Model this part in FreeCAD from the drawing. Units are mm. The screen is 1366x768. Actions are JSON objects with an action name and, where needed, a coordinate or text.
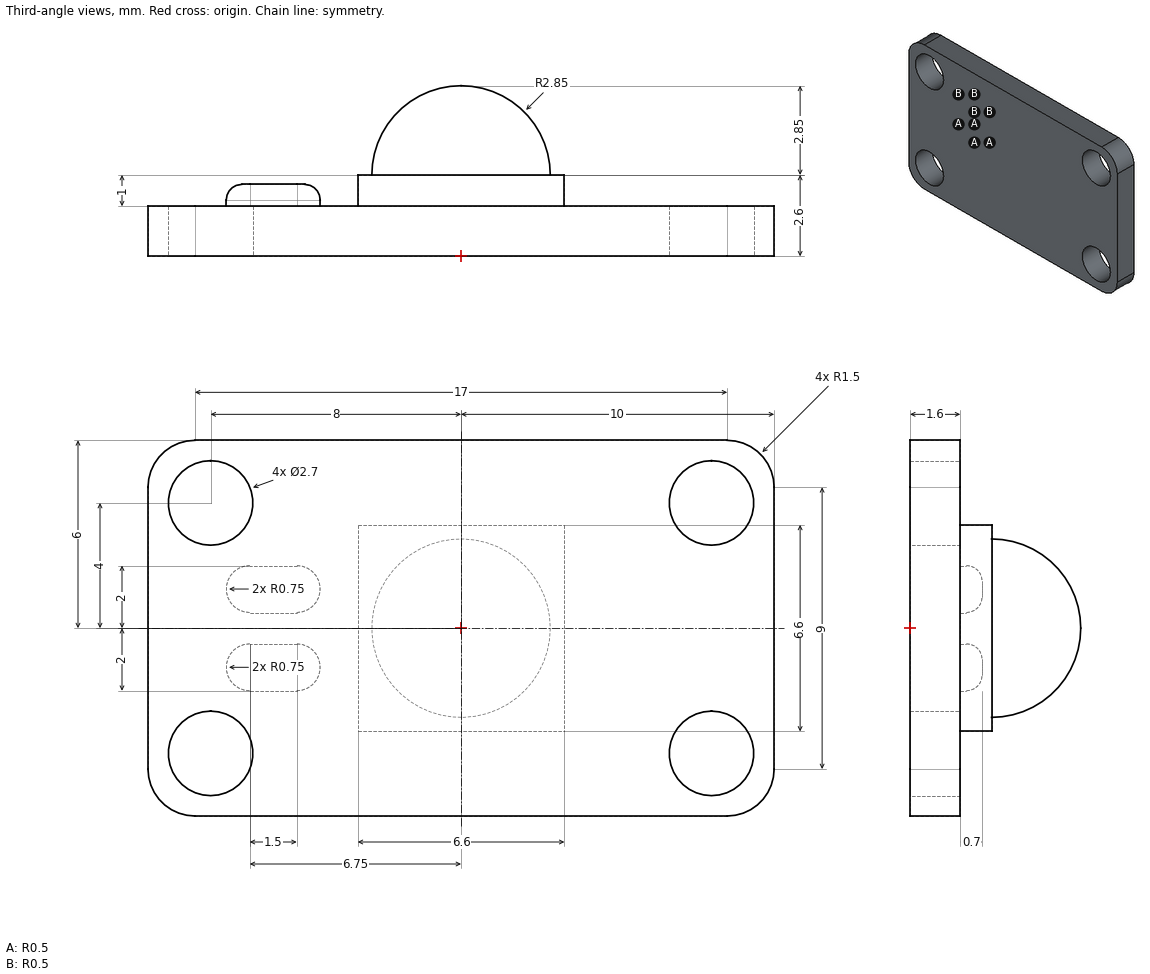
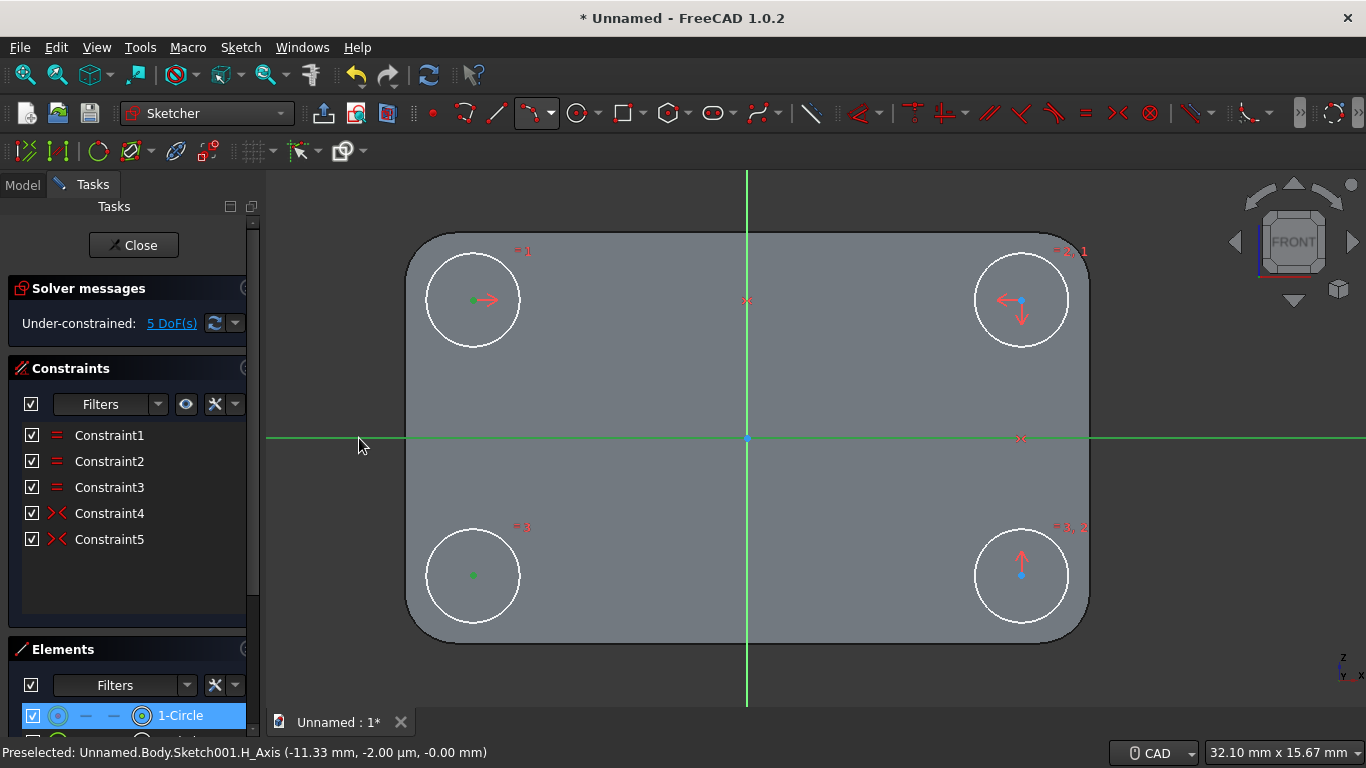
{"action": "left_click", "coordinate": [1118, 114]}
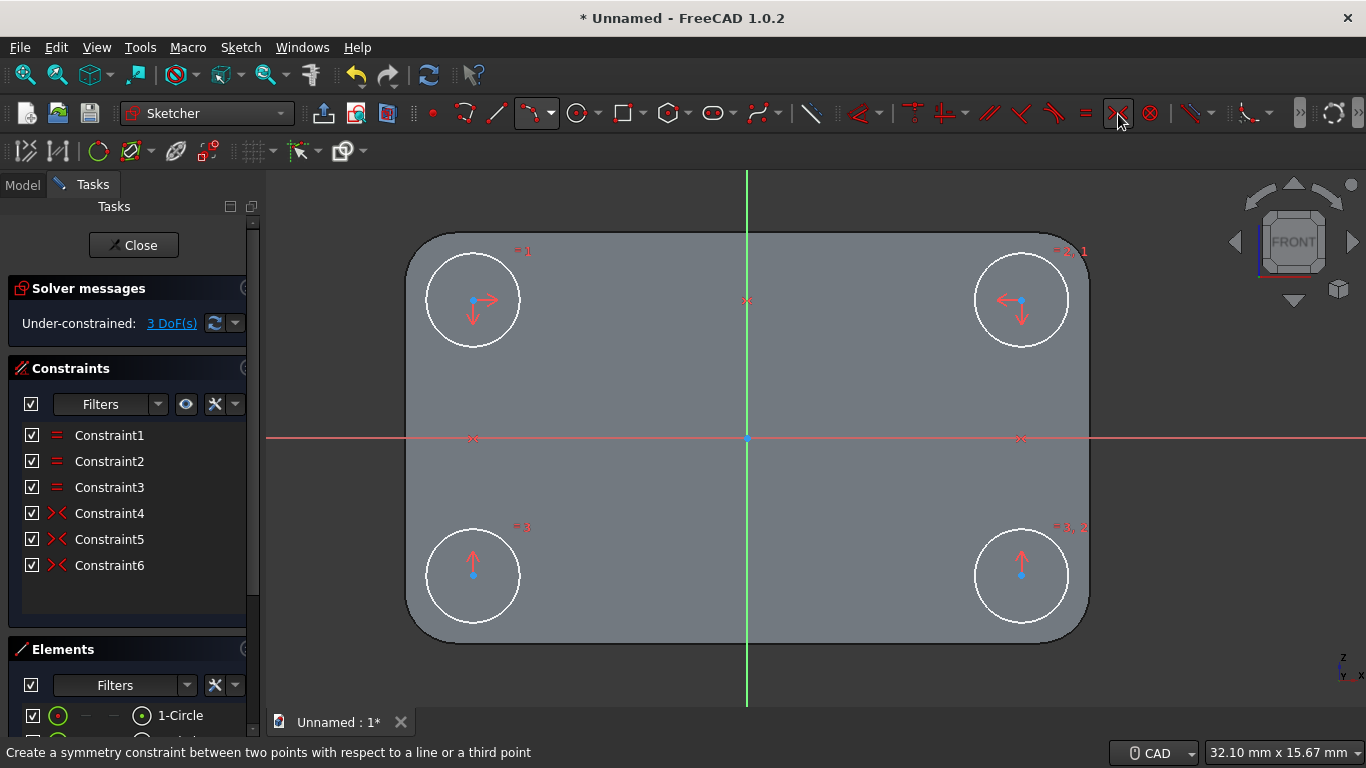
{"action": "left_click", "coordinate": [858, 114]}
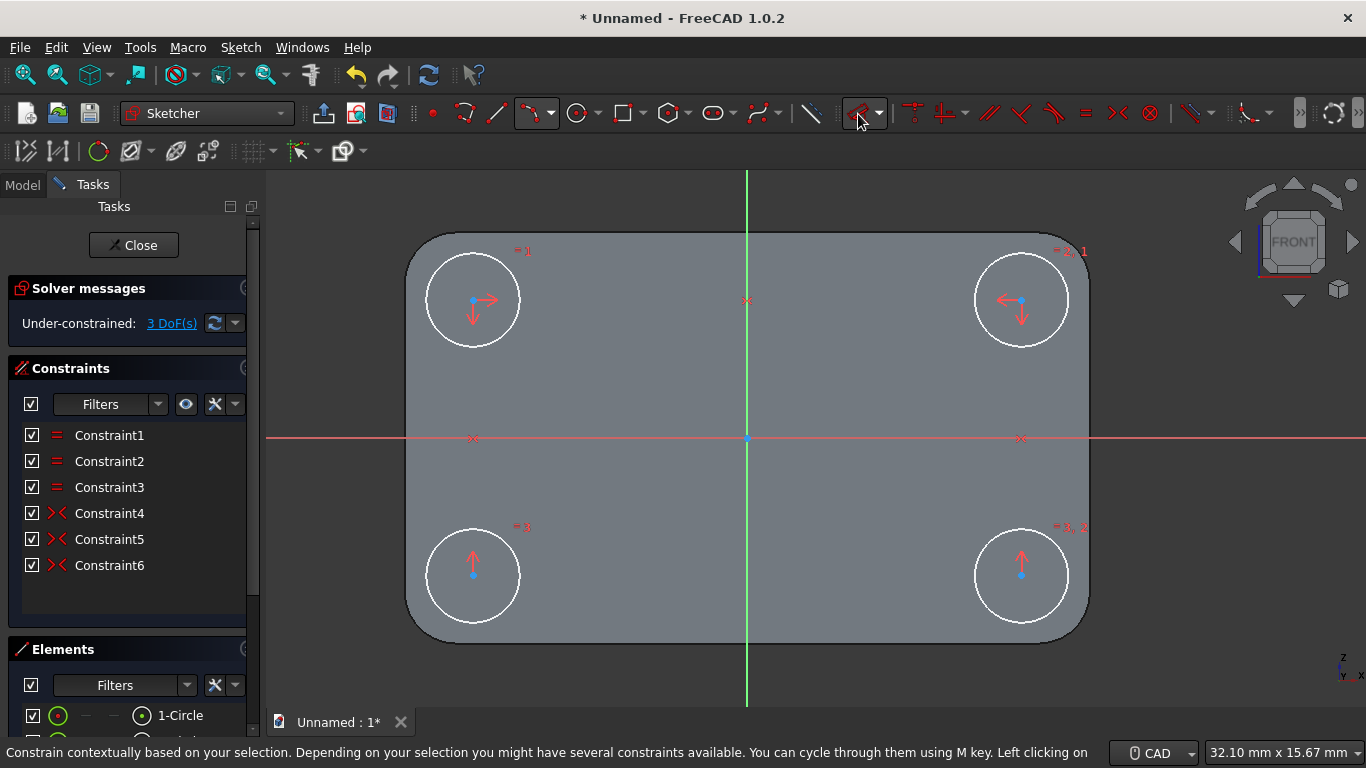
{"action": "left_click", "coordinate": [506, 267]}
{"action": "left_click", "coordinate": [529, 244]}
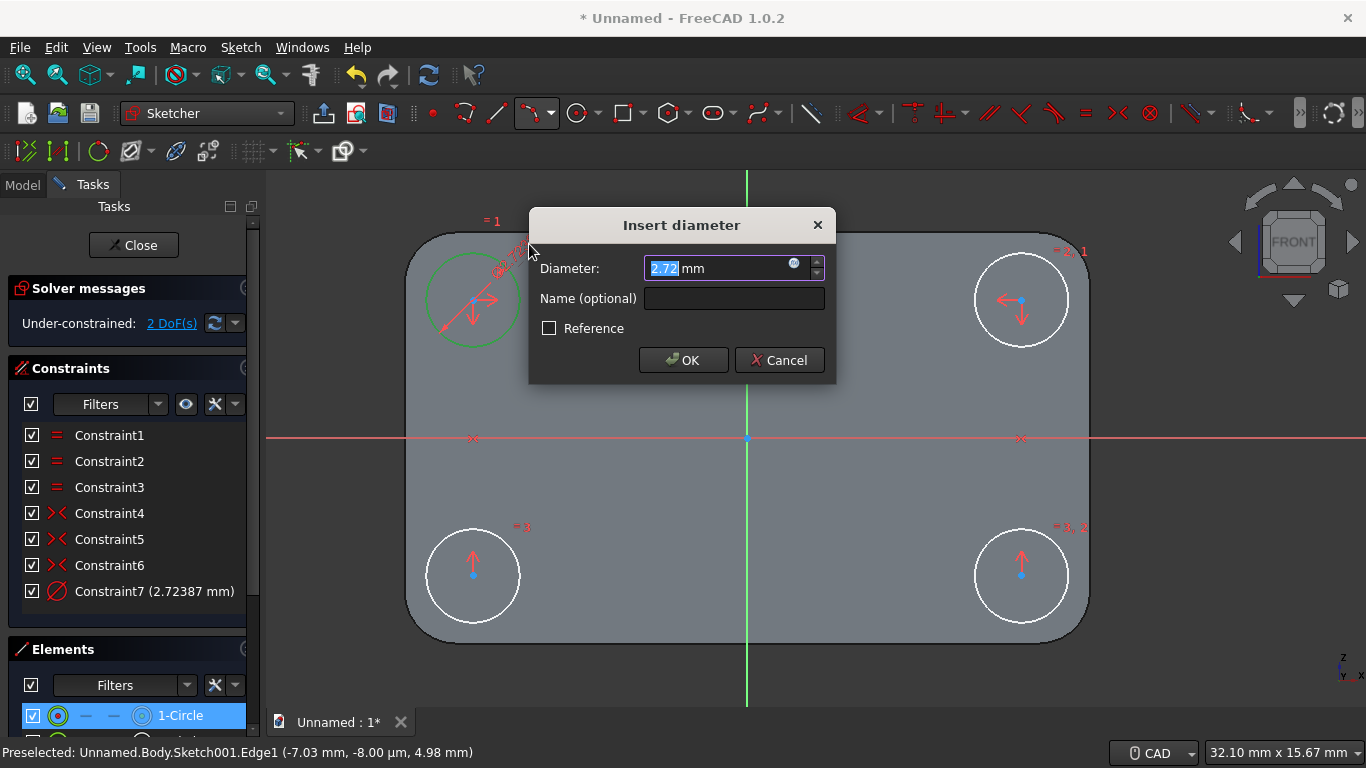
{"action": "type", "text": "2.7"}
{"action": "key", "text": "Return"}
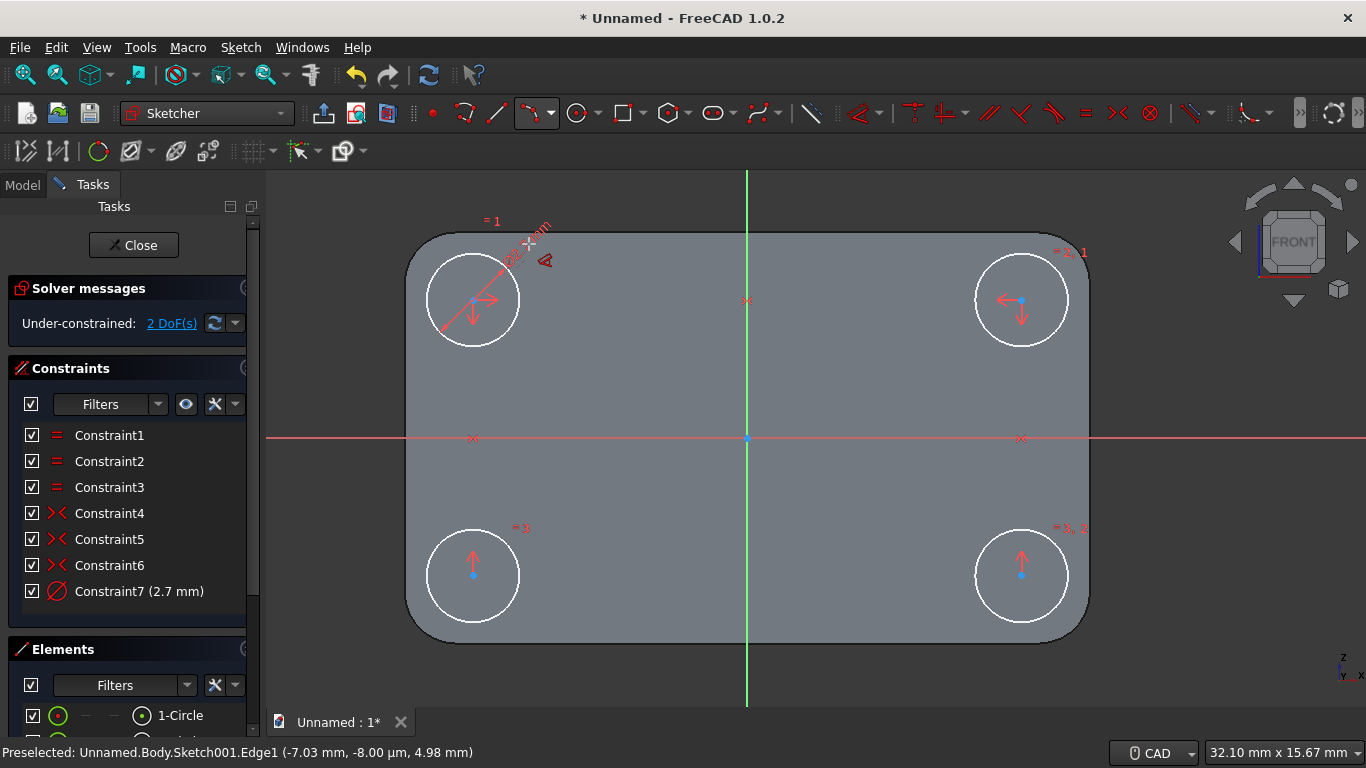
{"action": "left_click", "coordinate": [473, 300]}
{"action": "left_click", "coordinate": [610, 266]}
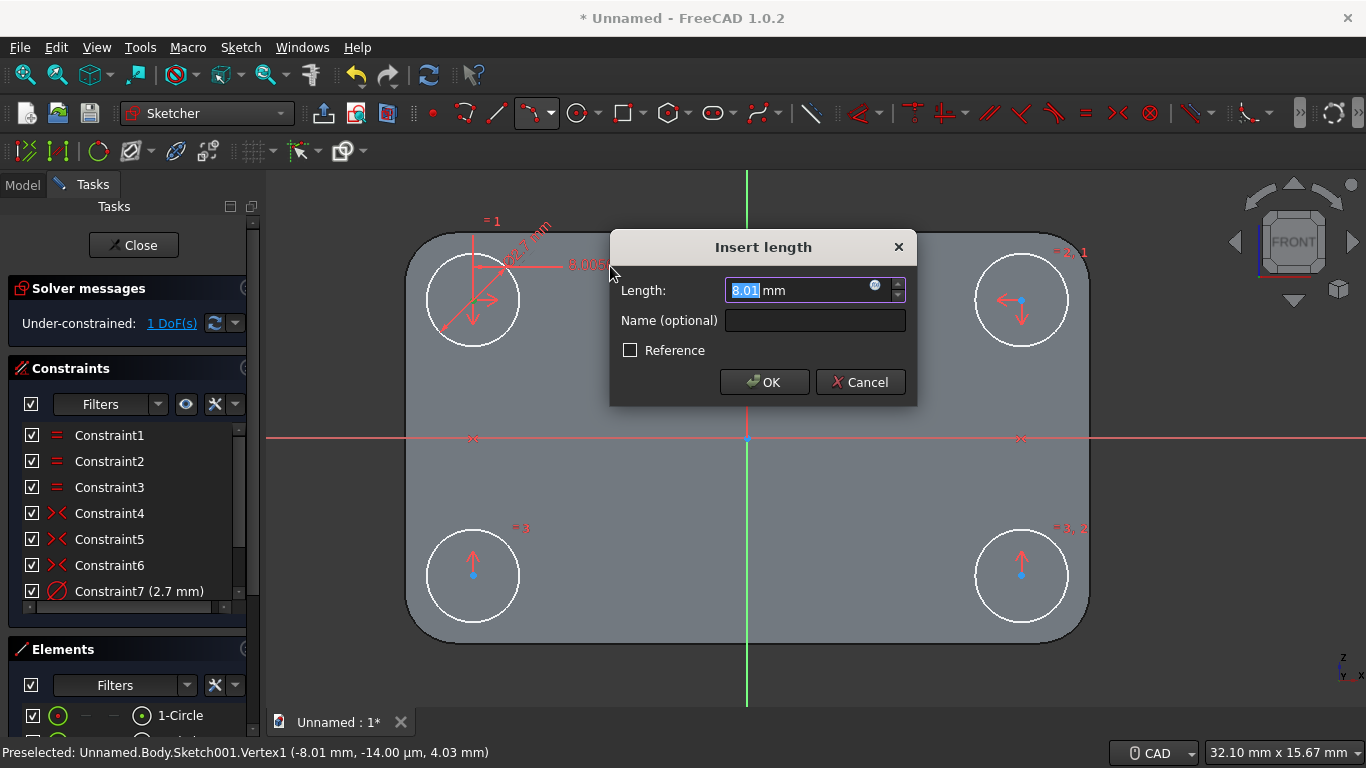
{"action": "type", "text": "8"}
{"action": "key", "text": "Return"}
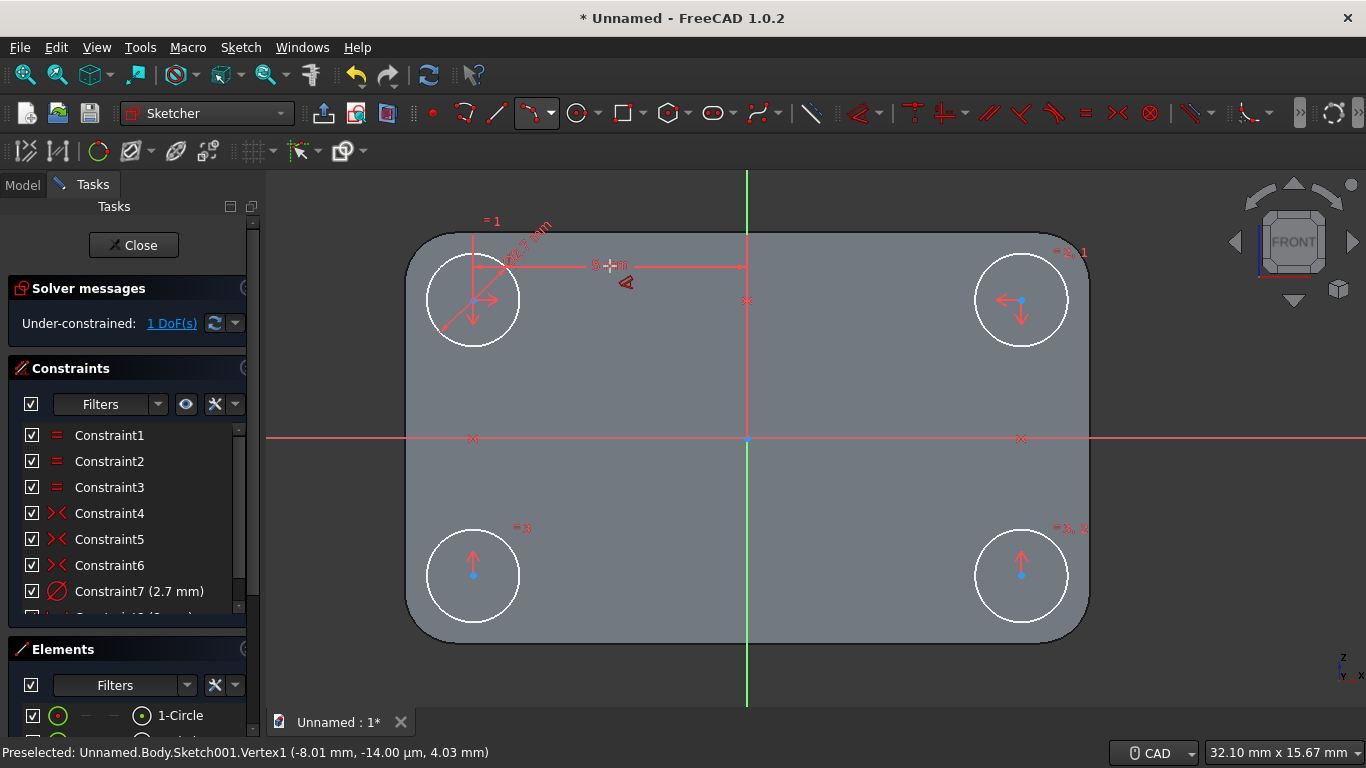
{"action": "left_click", "coordinate": [473, 300]}
{"action": "left_click", "coordinate": [439, 369]}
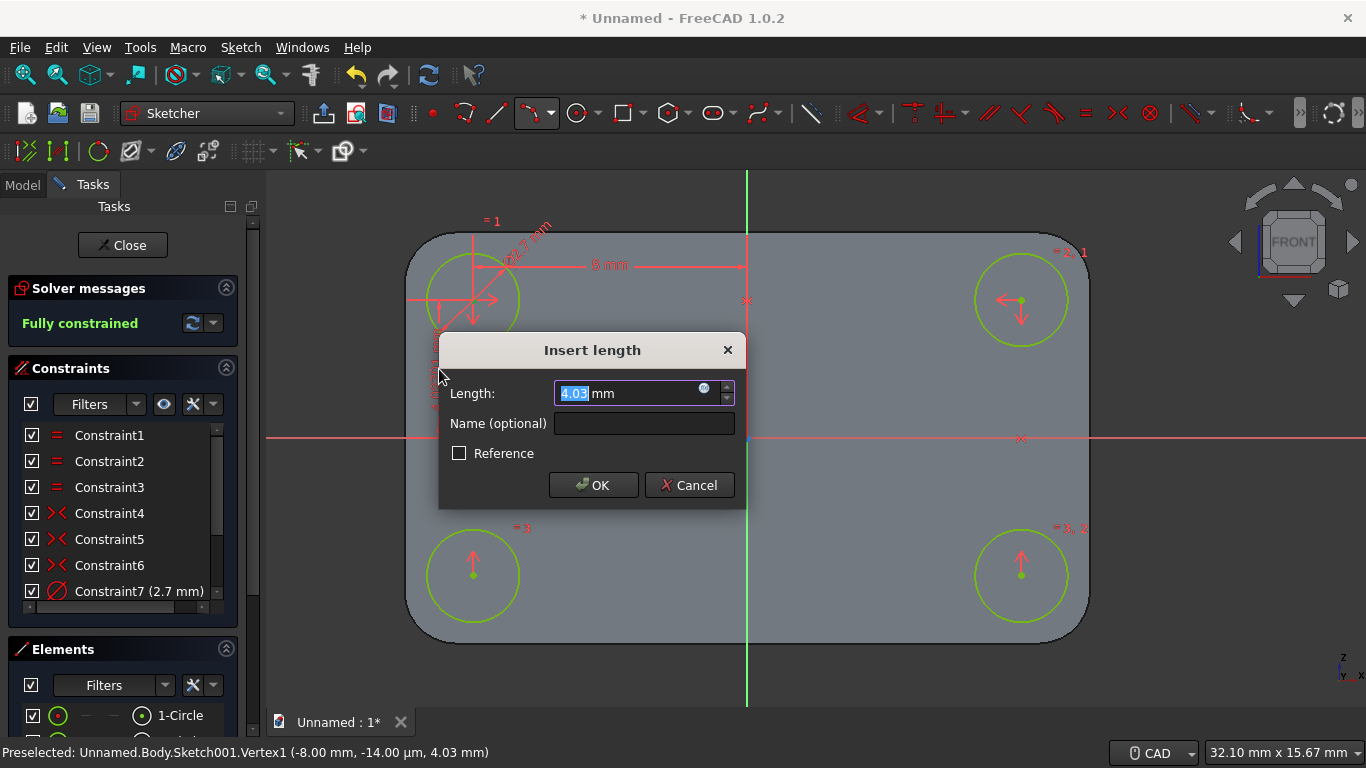
{"action": "type", "text": "4"}
{"action": "key", "text": "Return"}
{"action": "key", "text": "Escape"}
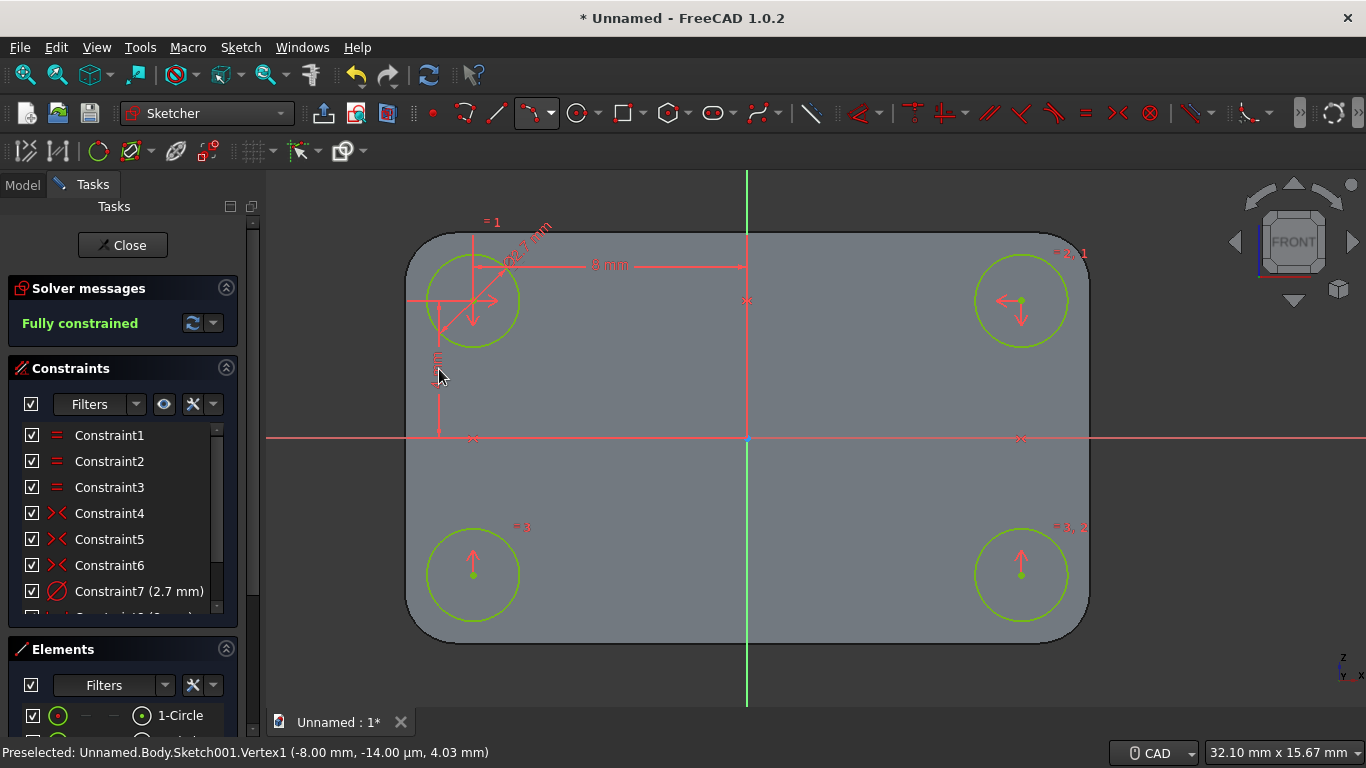
{"action": "left_click", "coordinate": [123, 245]}